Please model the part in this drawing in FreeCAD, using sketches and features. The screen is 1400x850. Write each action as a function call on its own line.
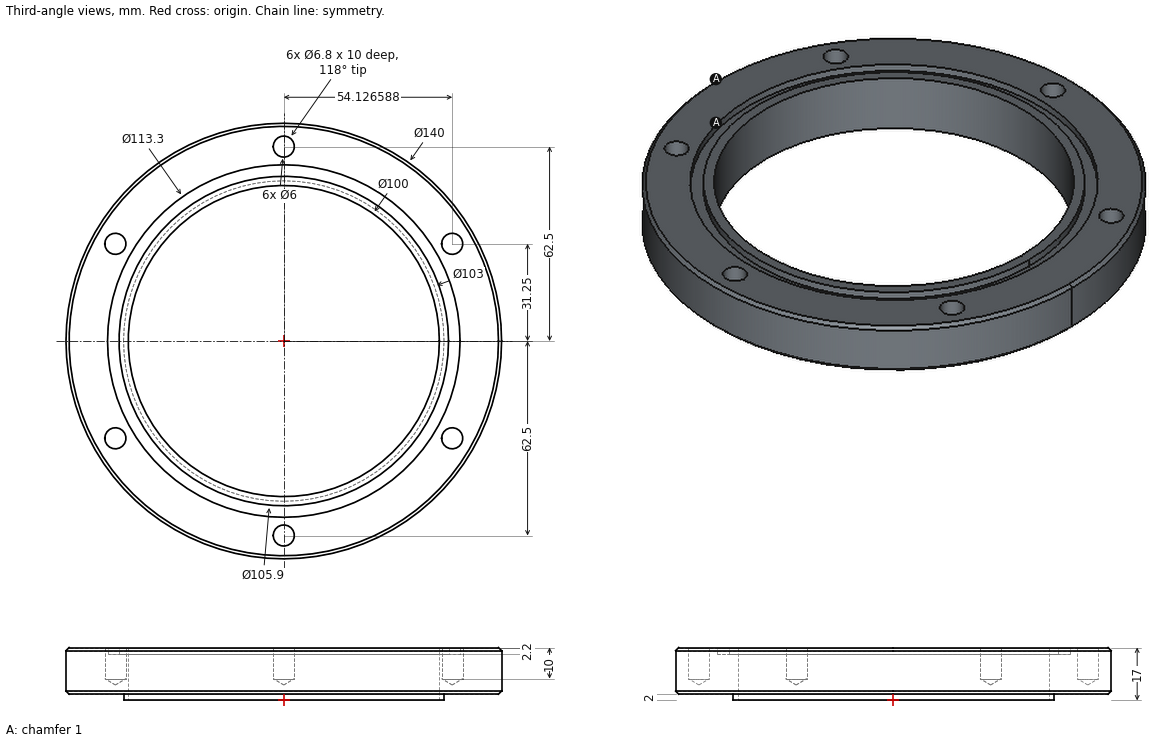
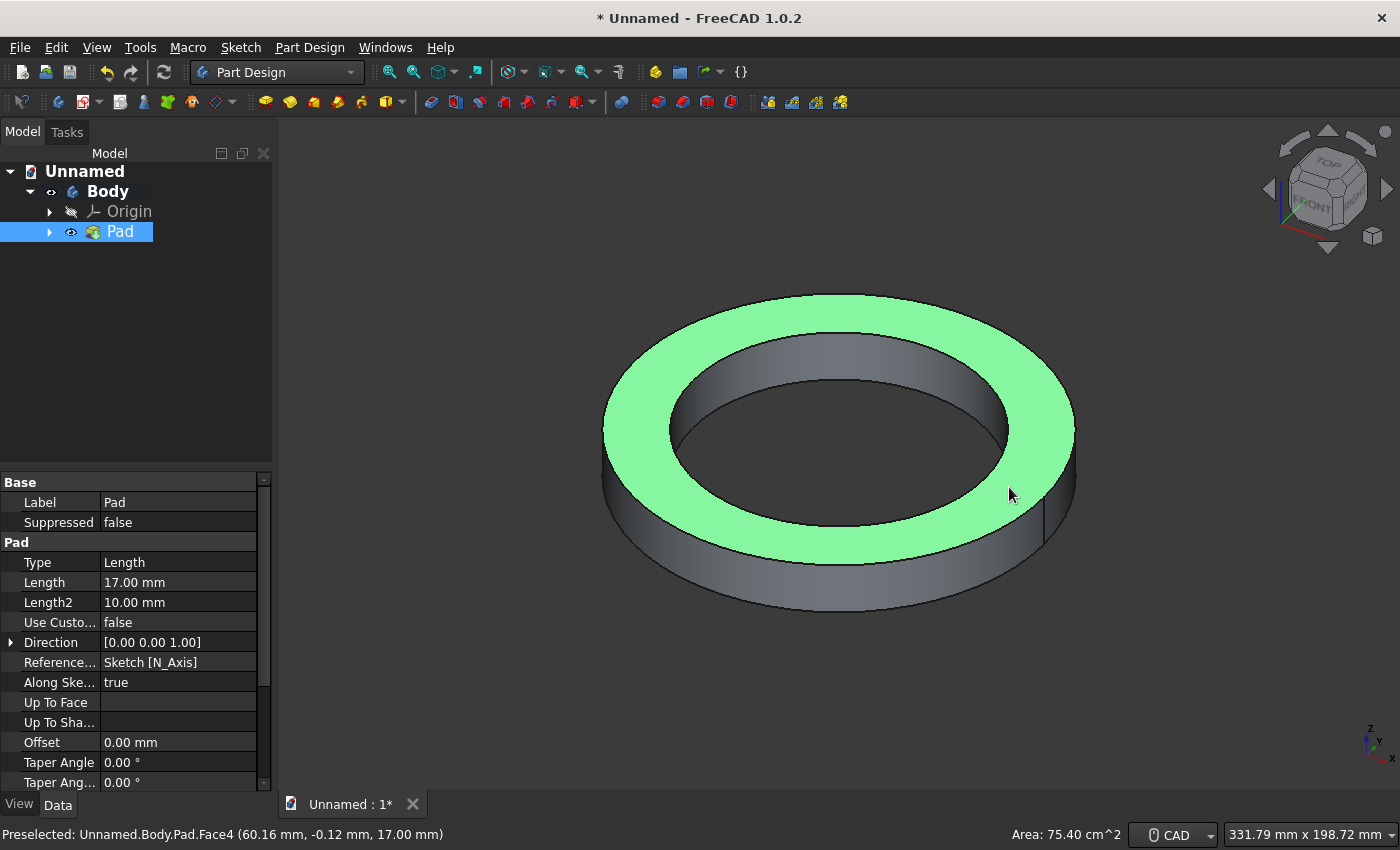
click(84, 102)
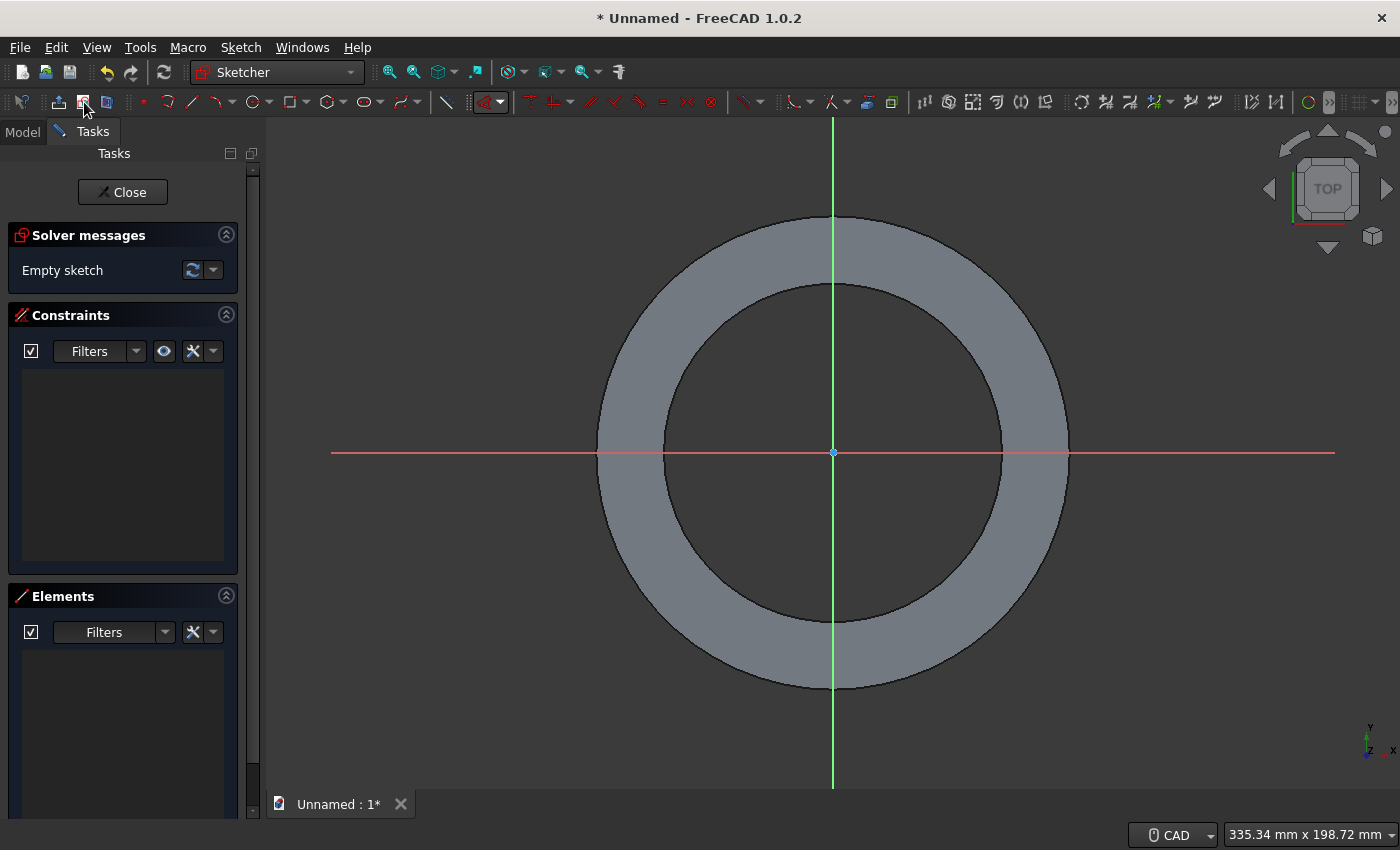
click(254, 102)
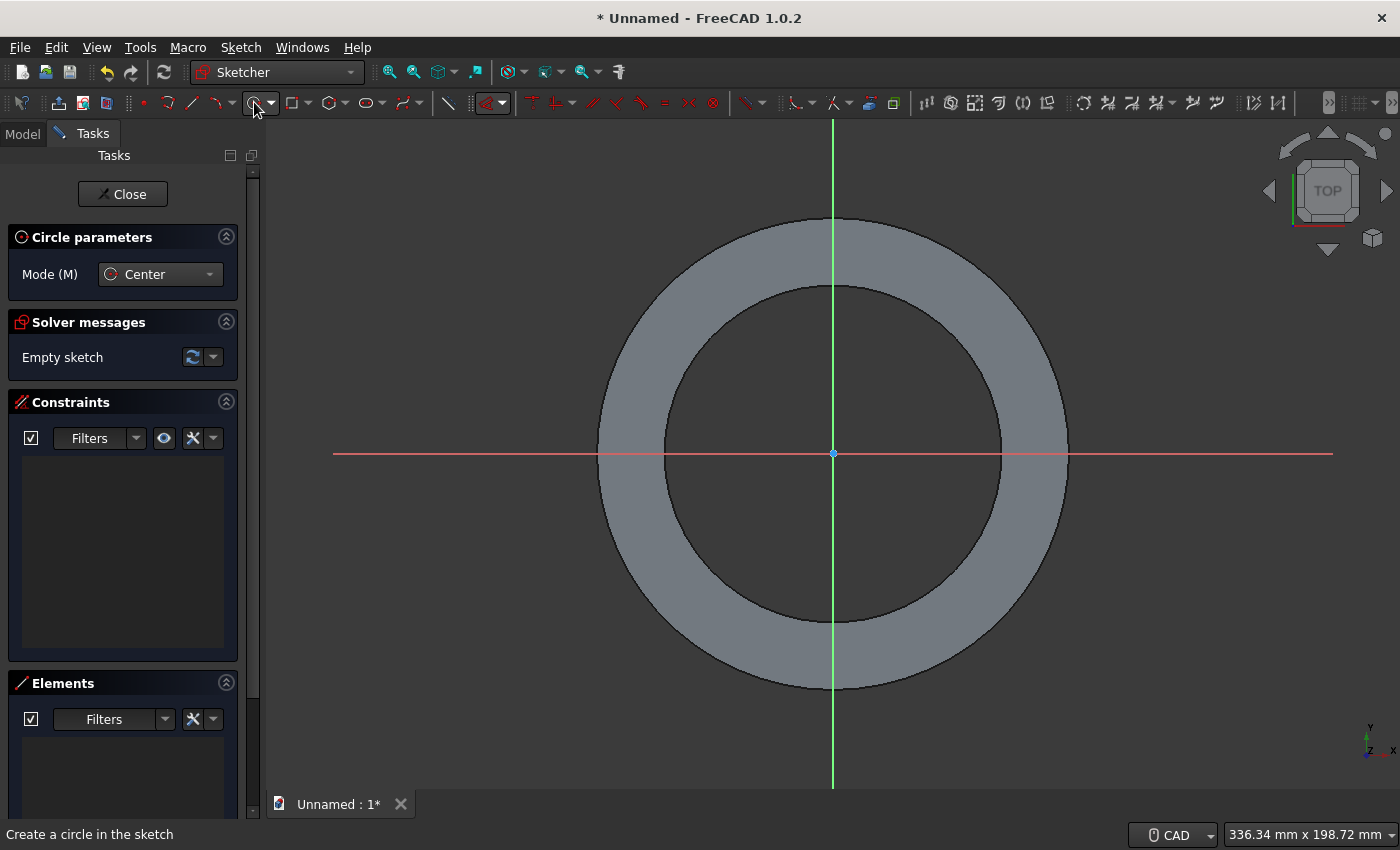
click(833, 454)
move(968, 319)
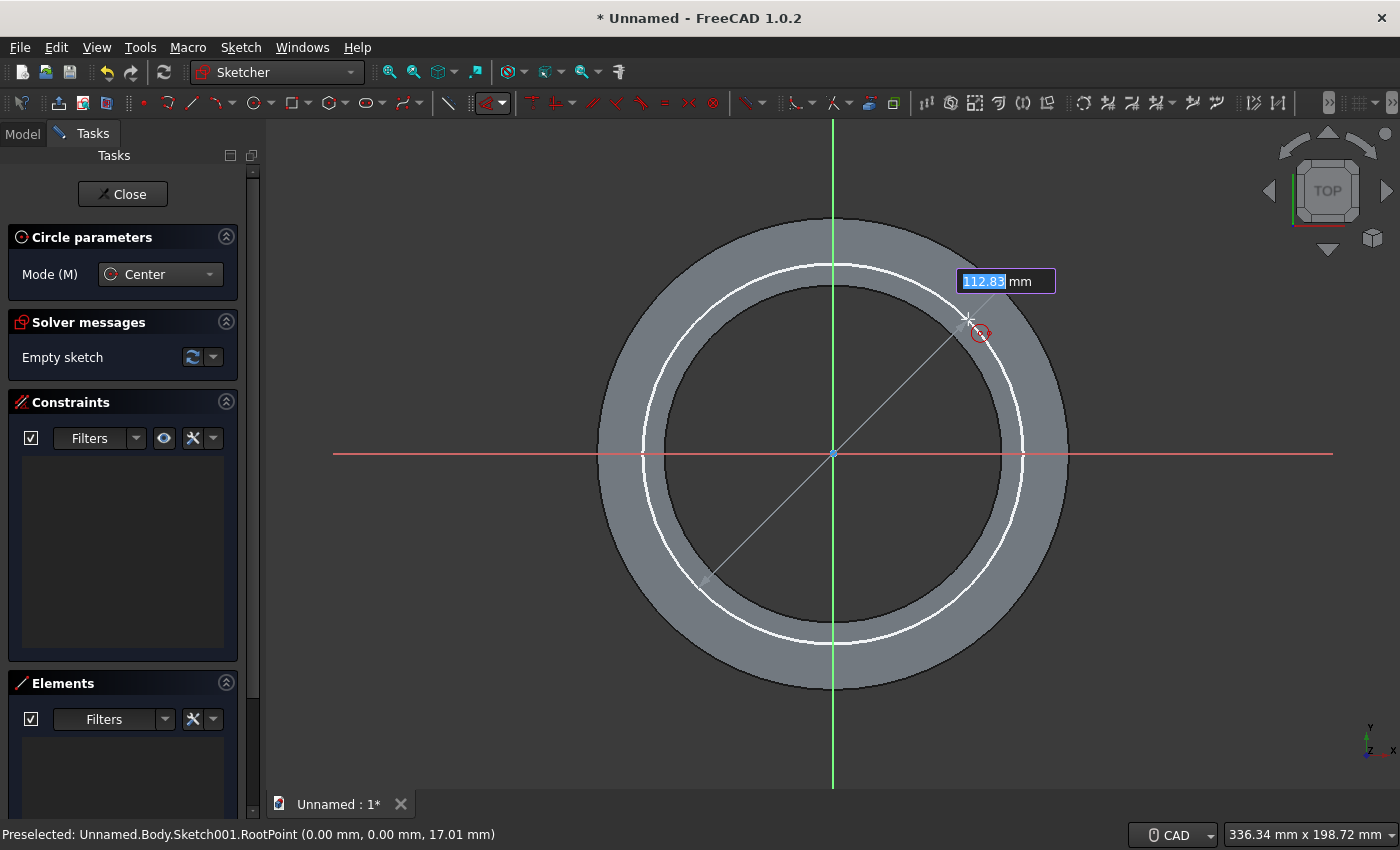
text(113.3)
key(Return)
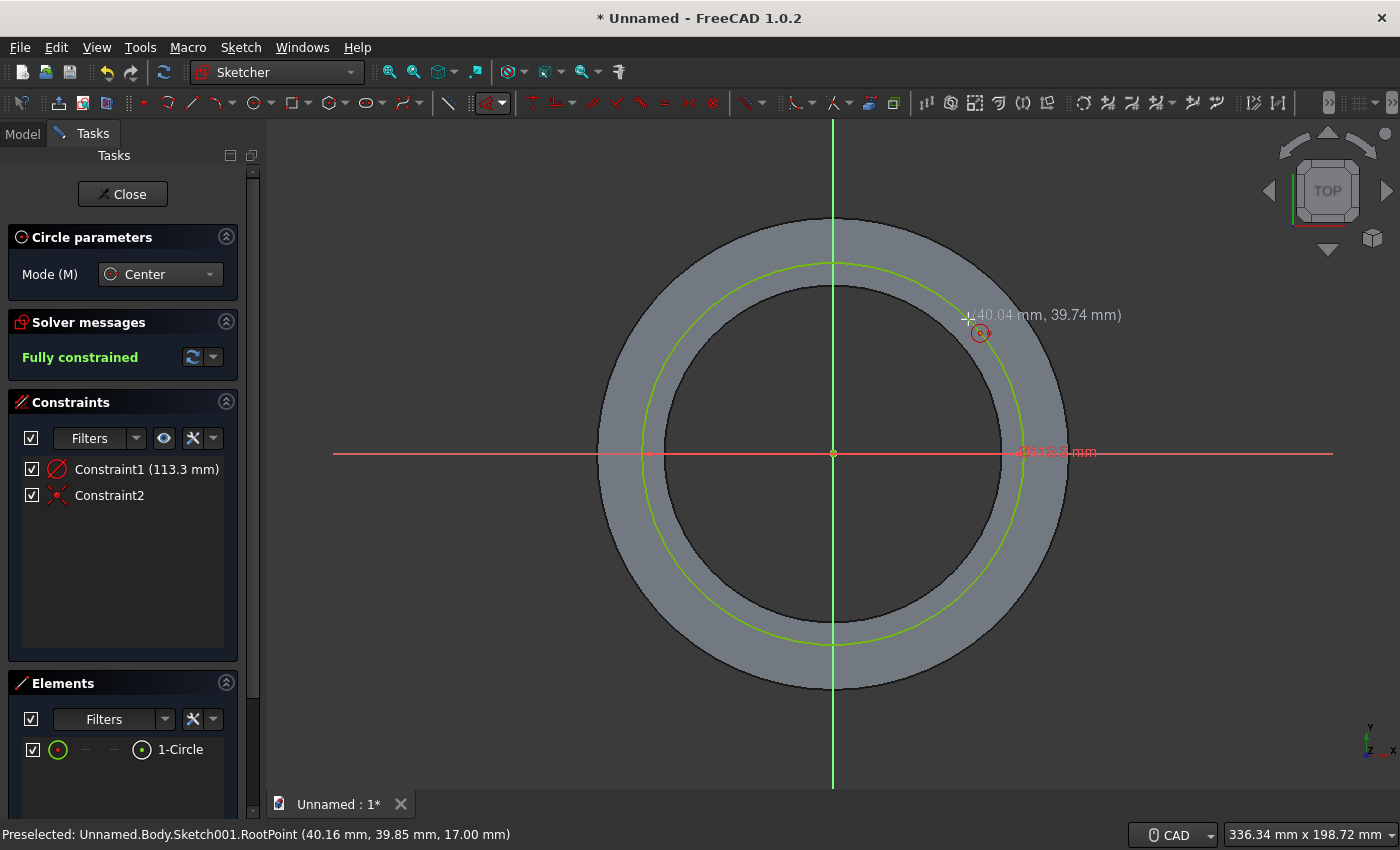
click(833, 454)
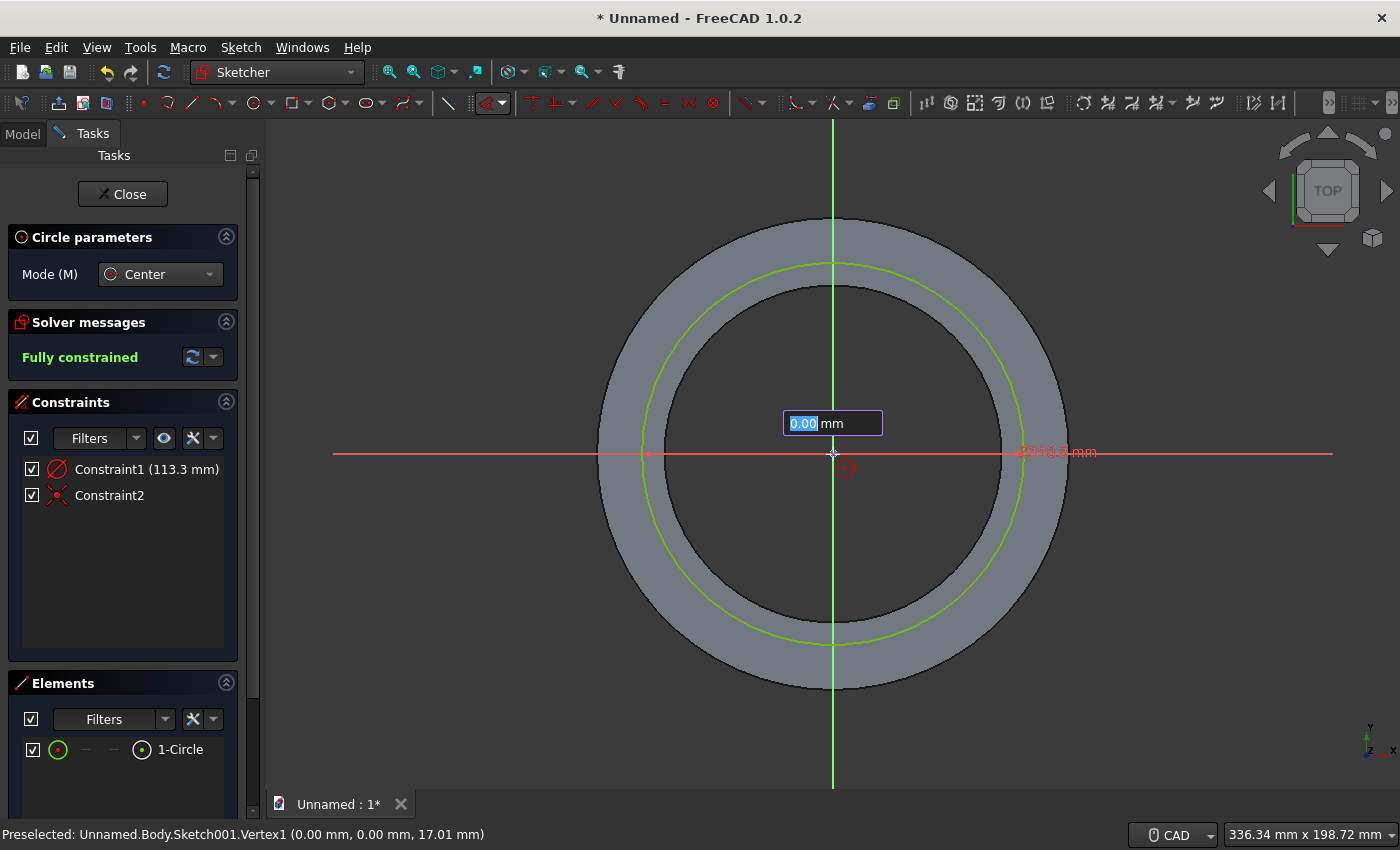
scroll(959, 328, up, 2)
move(959, 327)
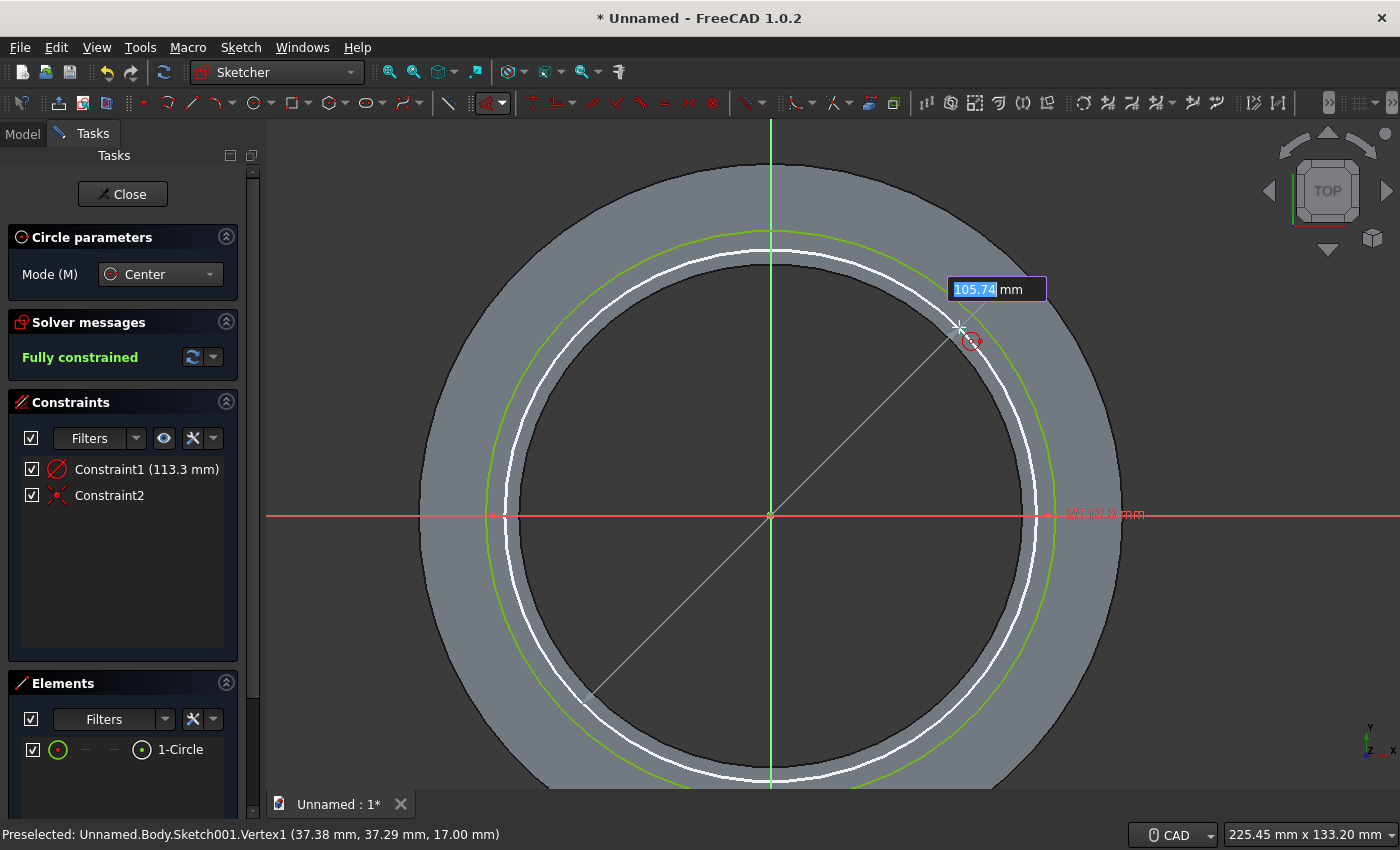
text(105.9)
key(Return)
key(Escape)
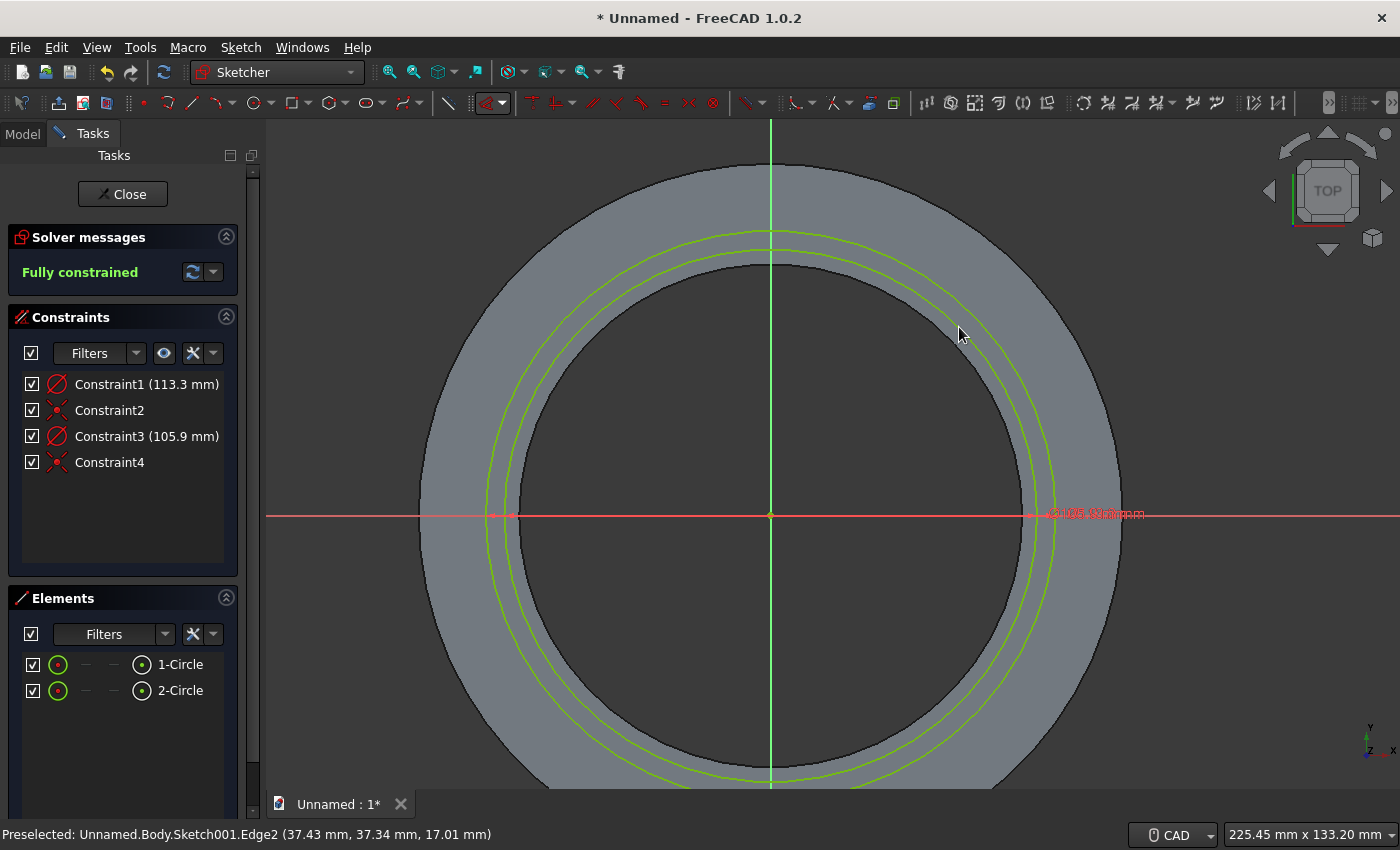
click(123, 194)